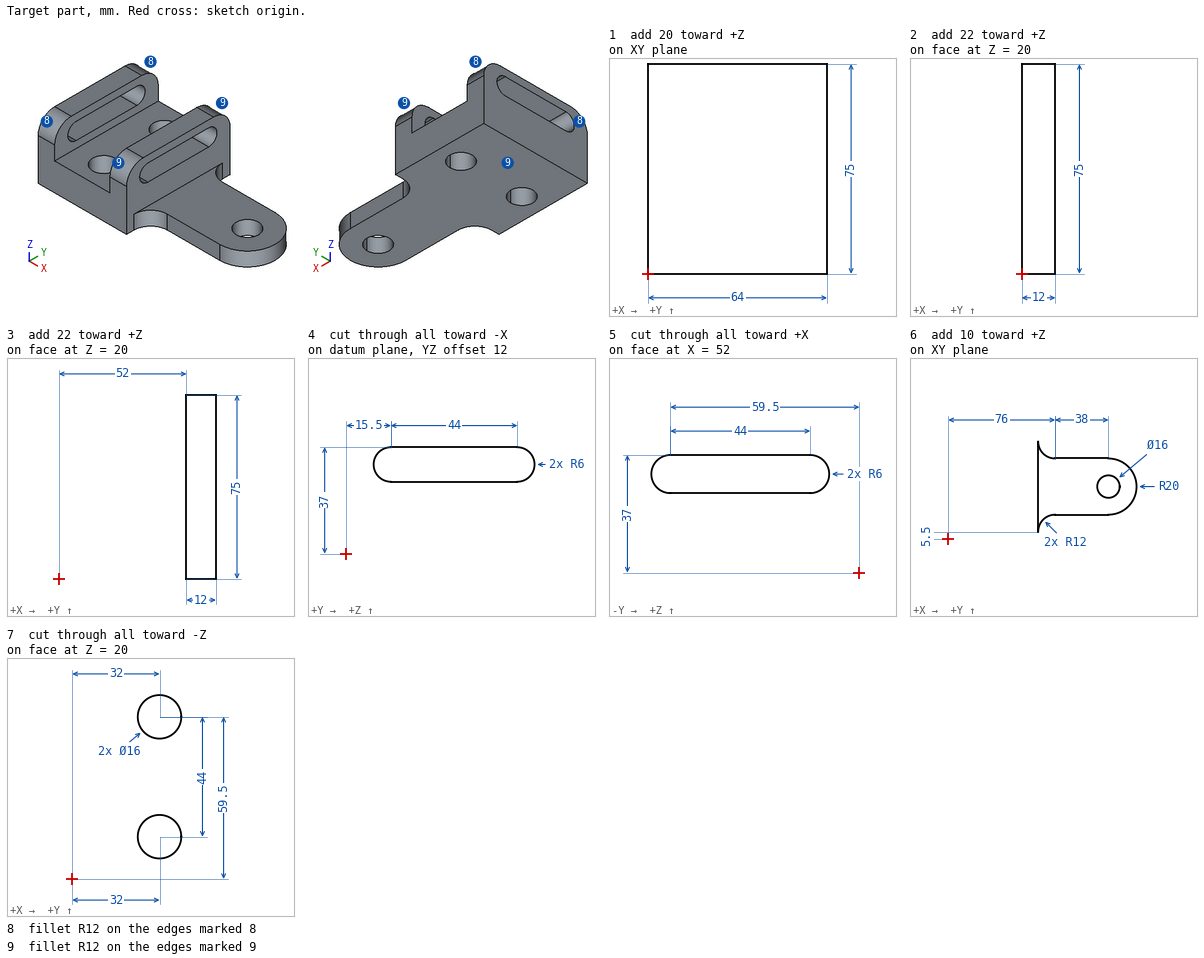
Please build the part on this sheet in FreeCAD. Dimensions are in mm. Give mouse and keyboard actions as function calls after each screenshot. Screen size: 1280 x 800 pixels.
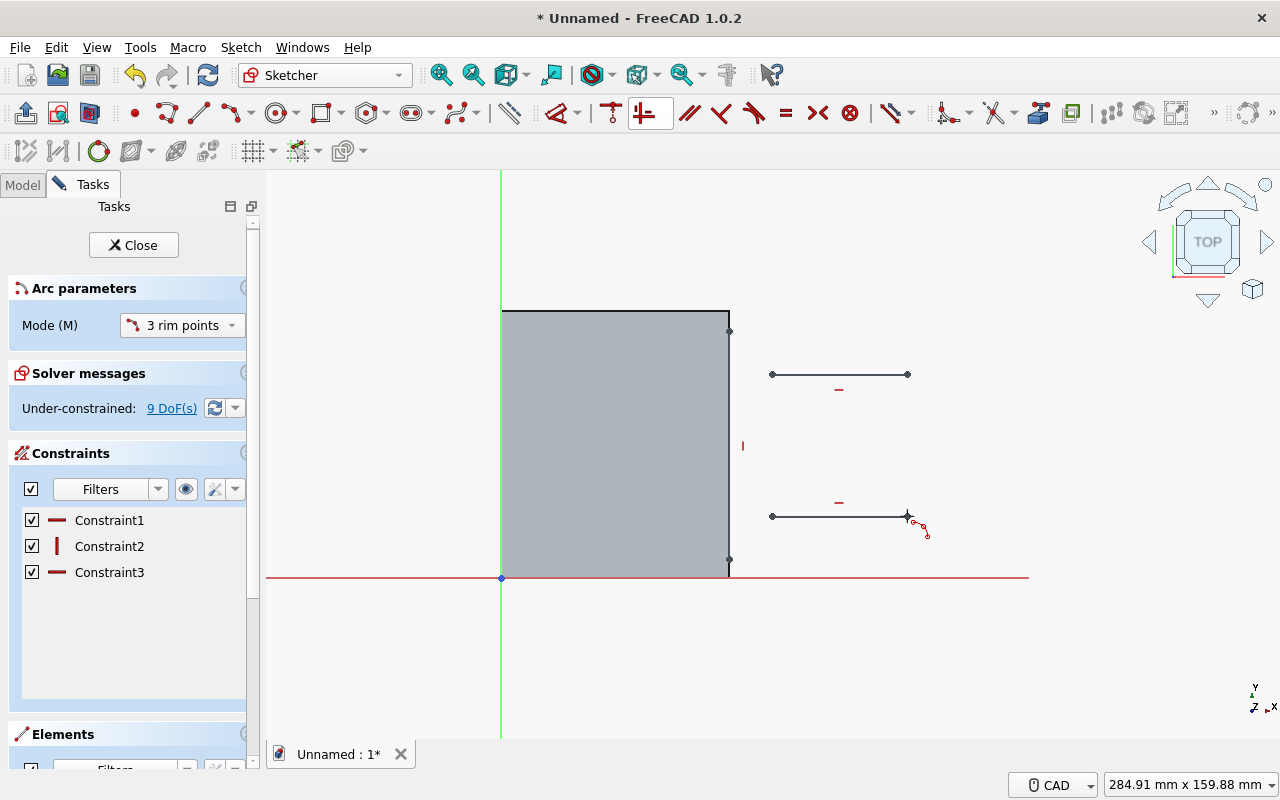
click(772, 375)
click(729, 332)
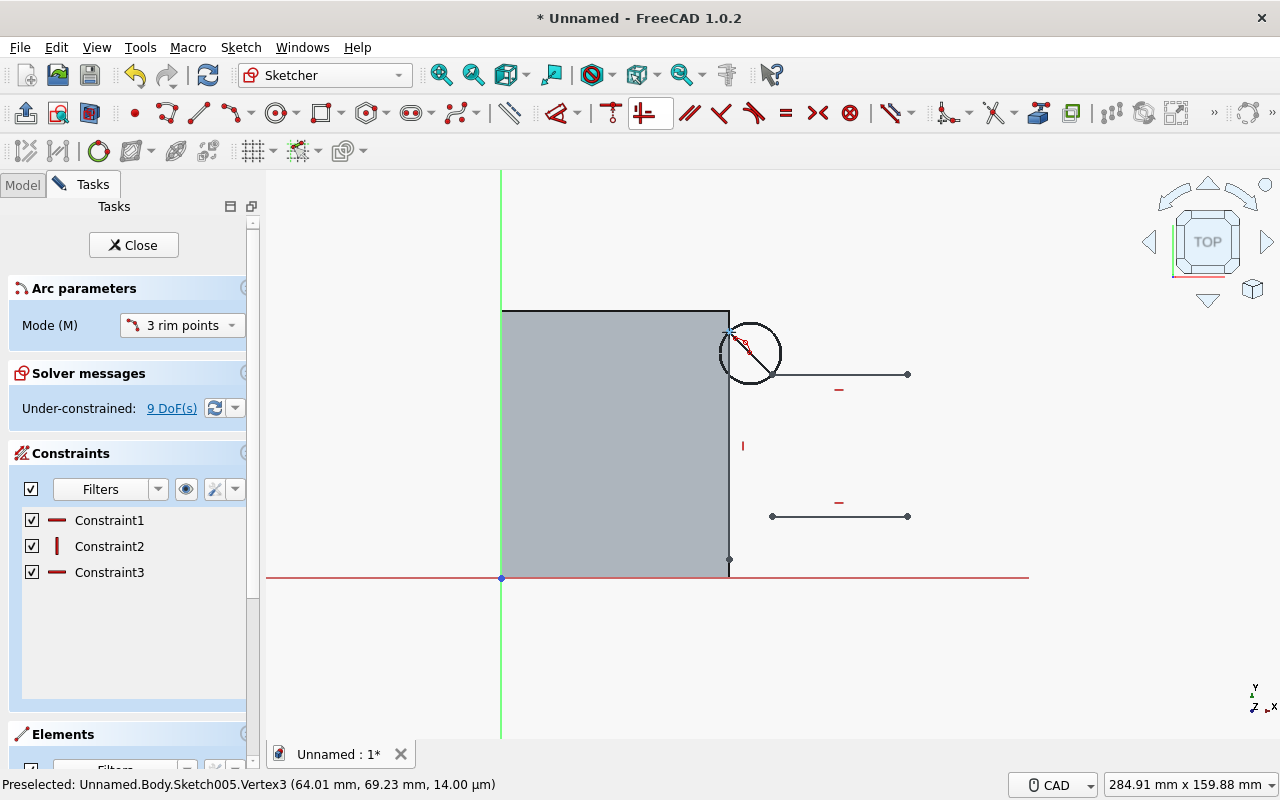
scroll(741, 361, up, 2)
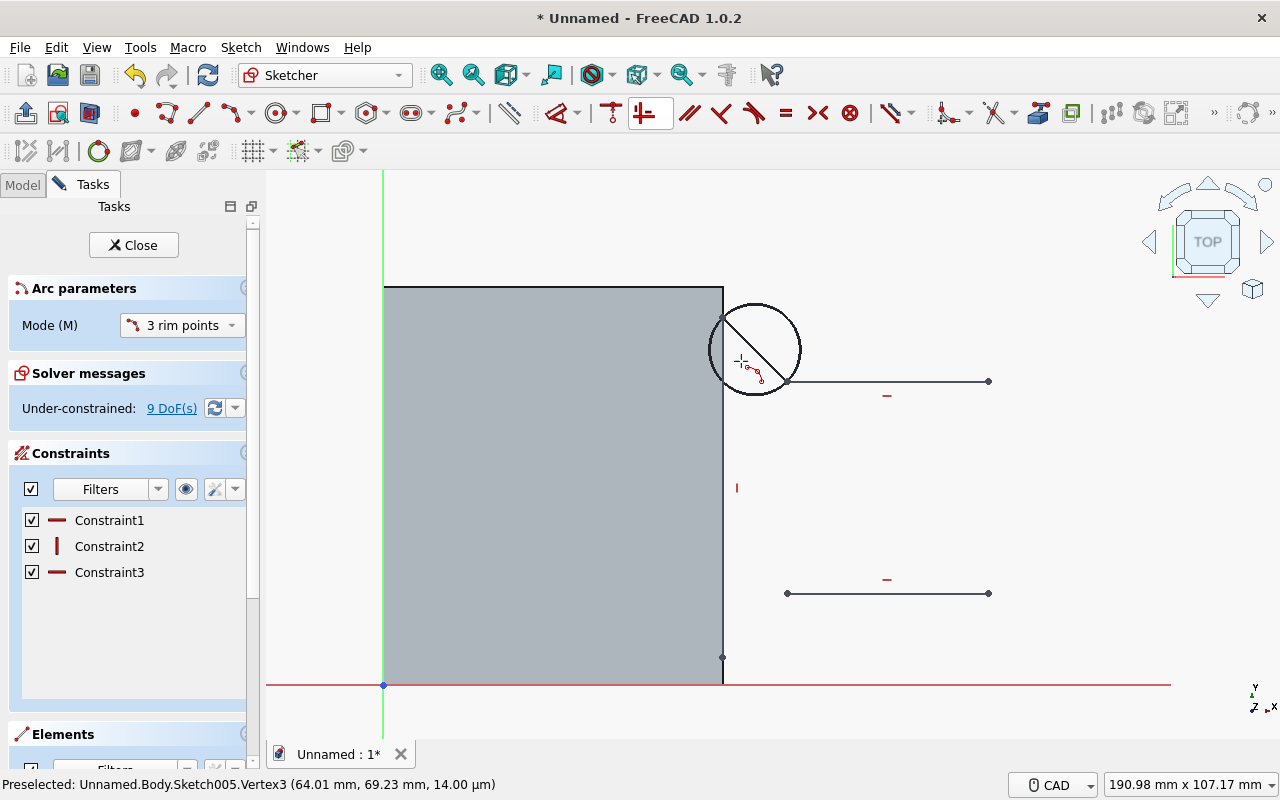
click(741, 361)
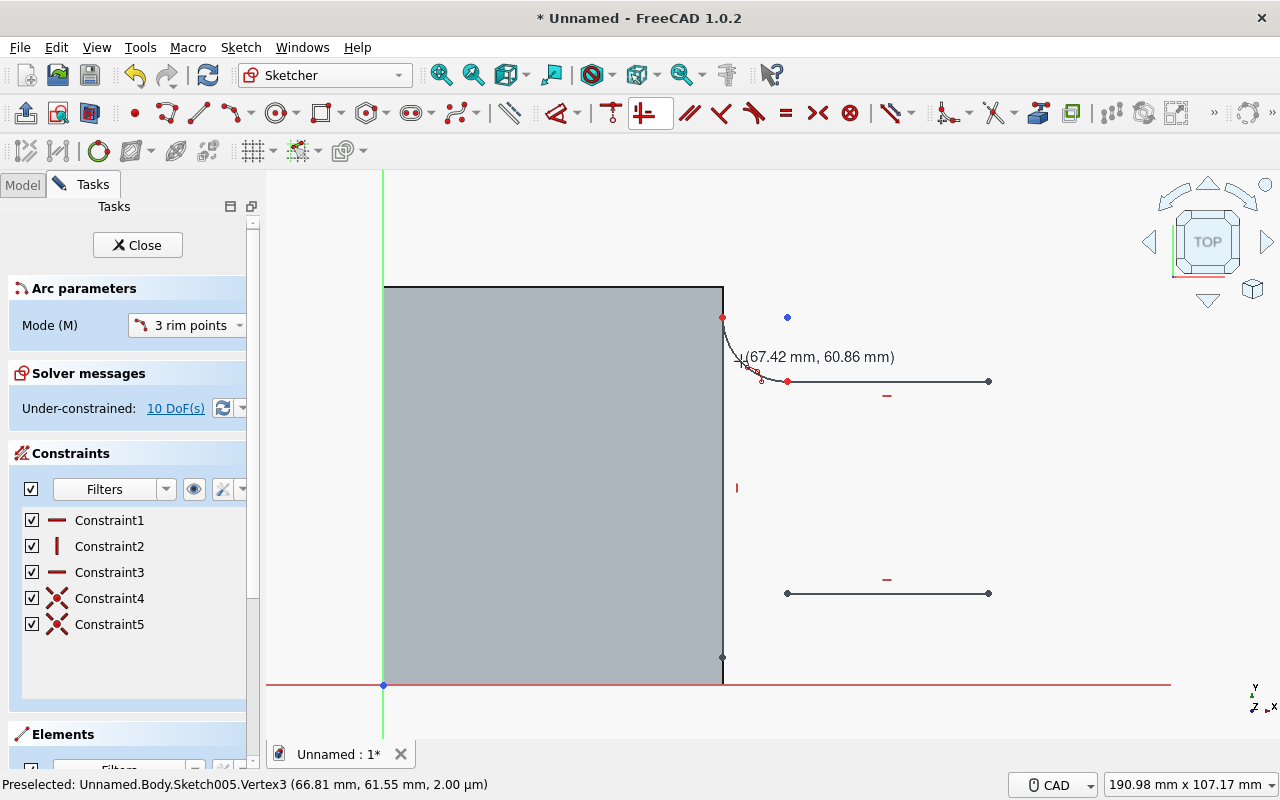
click(723, 658)
click(787, 594)
click(741, 611)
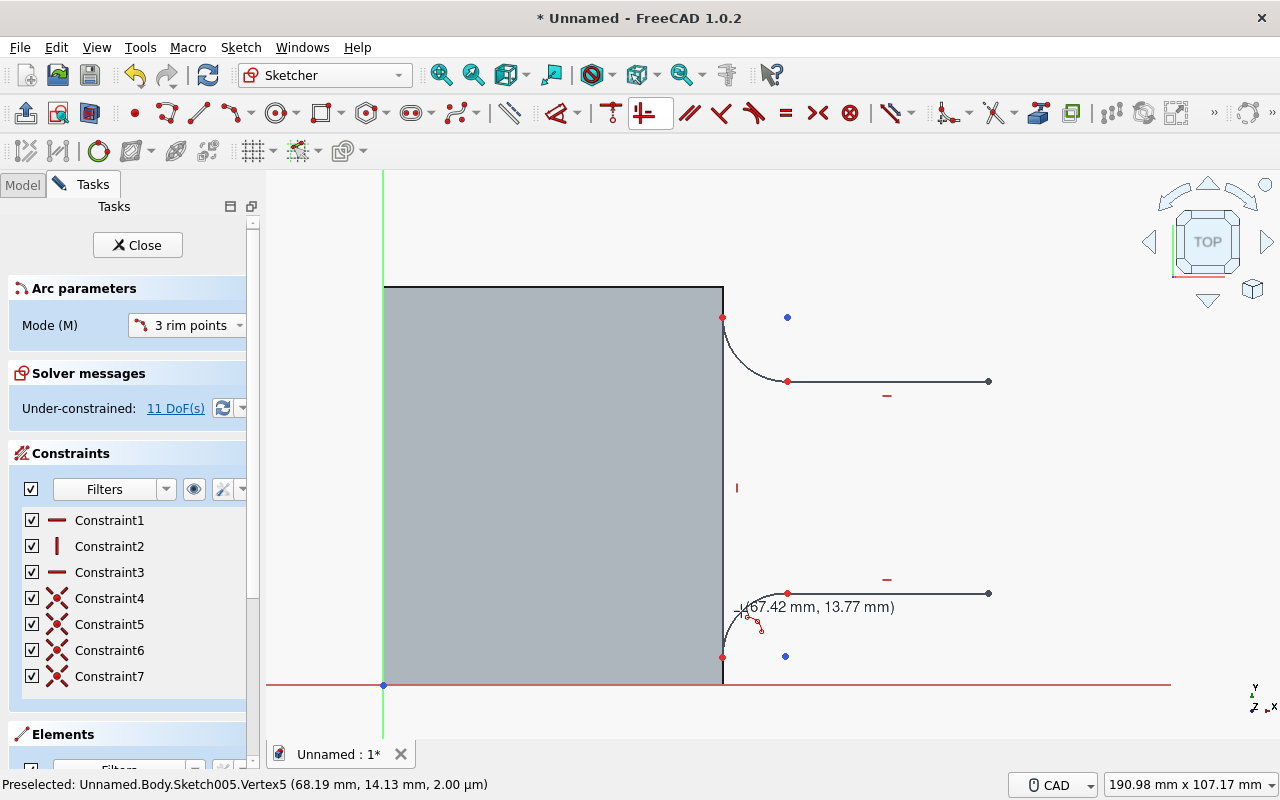
click(988, 594)
click(988, 382)
click(1094, 486)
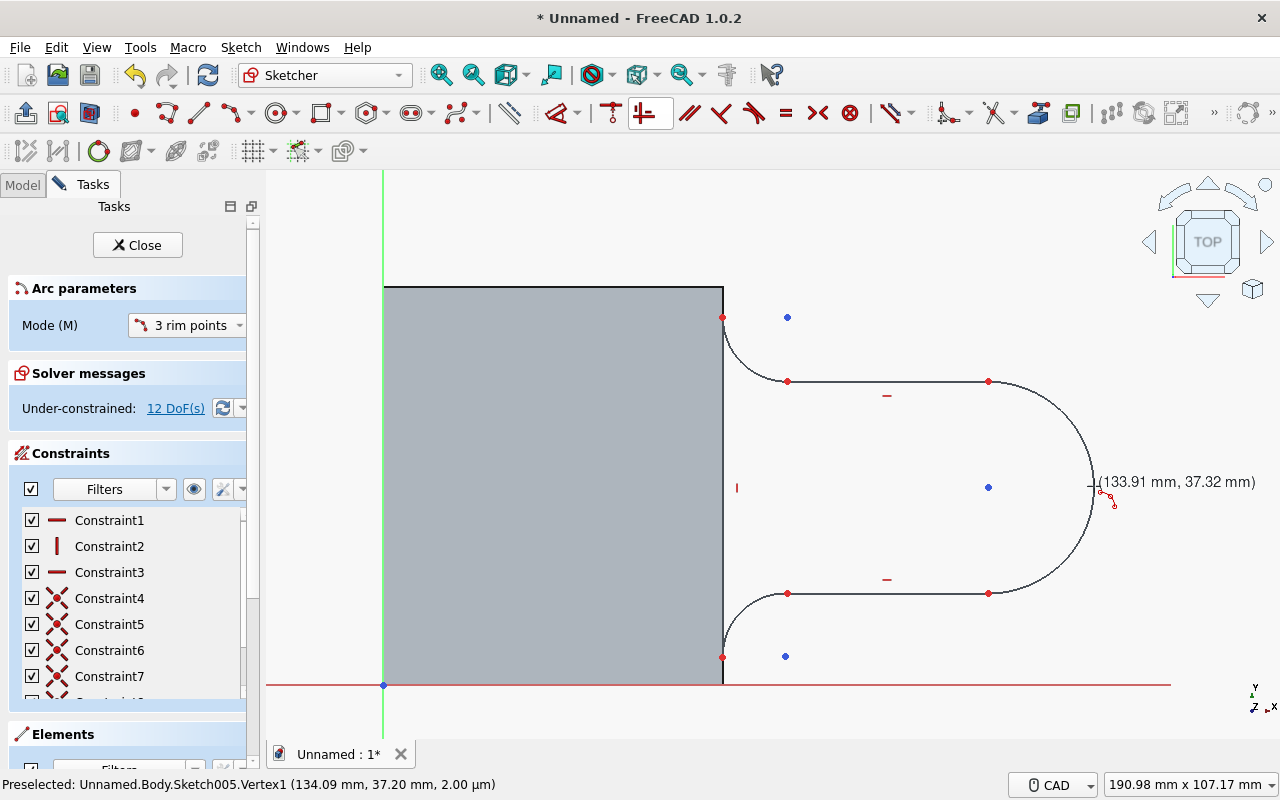
click(276, 114)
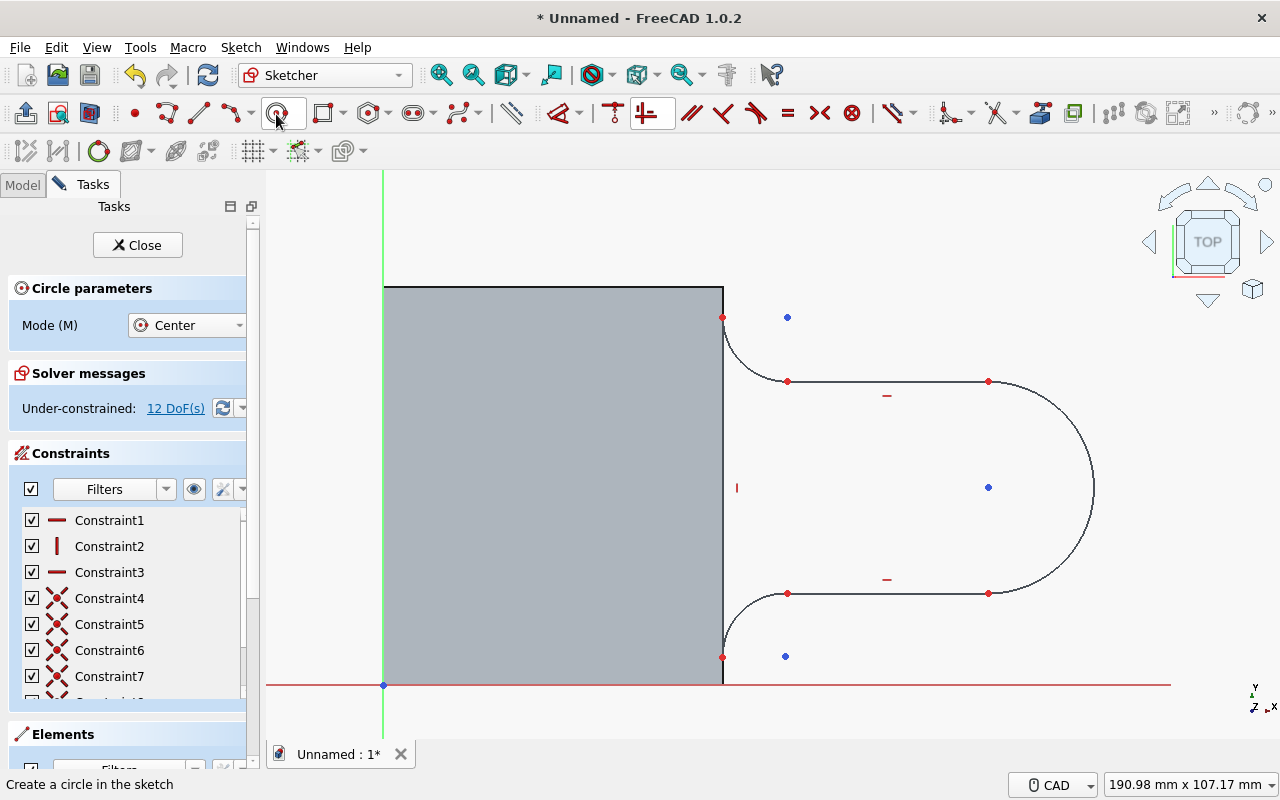
click(988, 486)
click(1018, 456)
key(Escape)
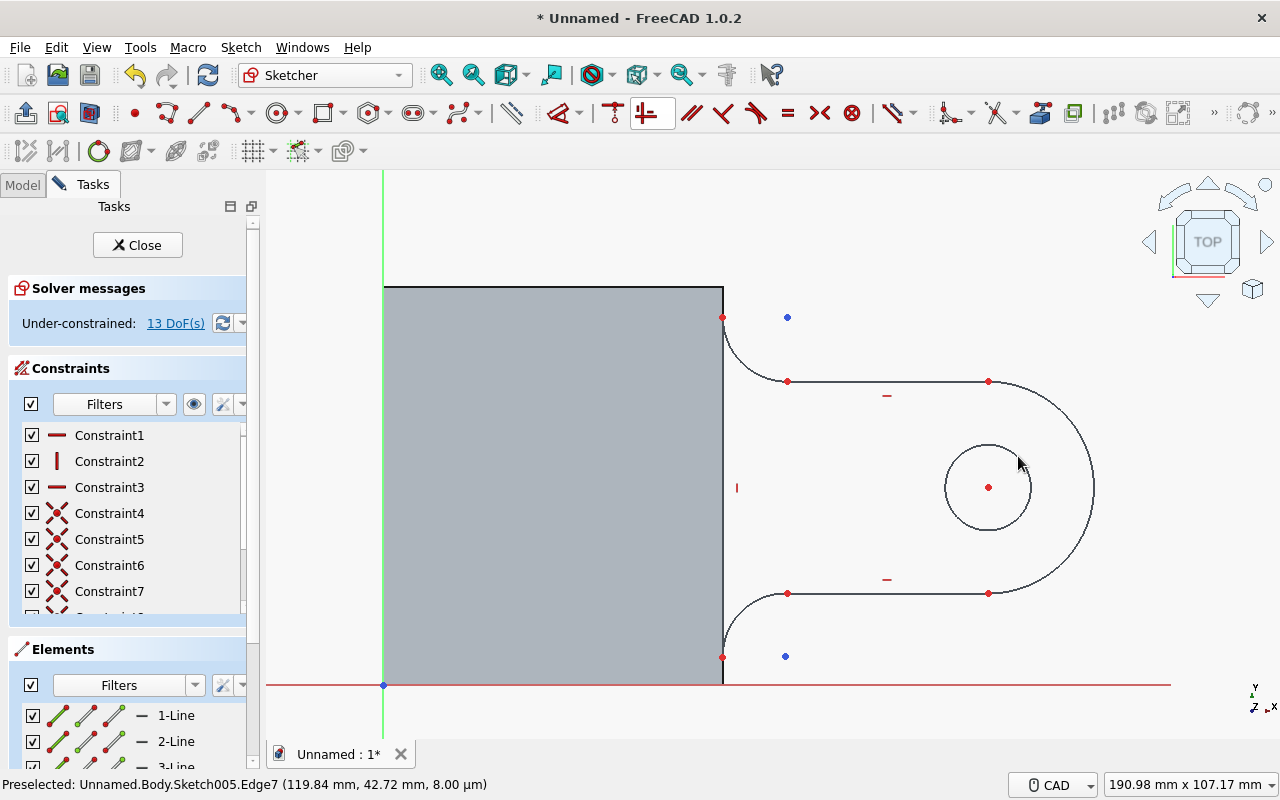
click(928, 382)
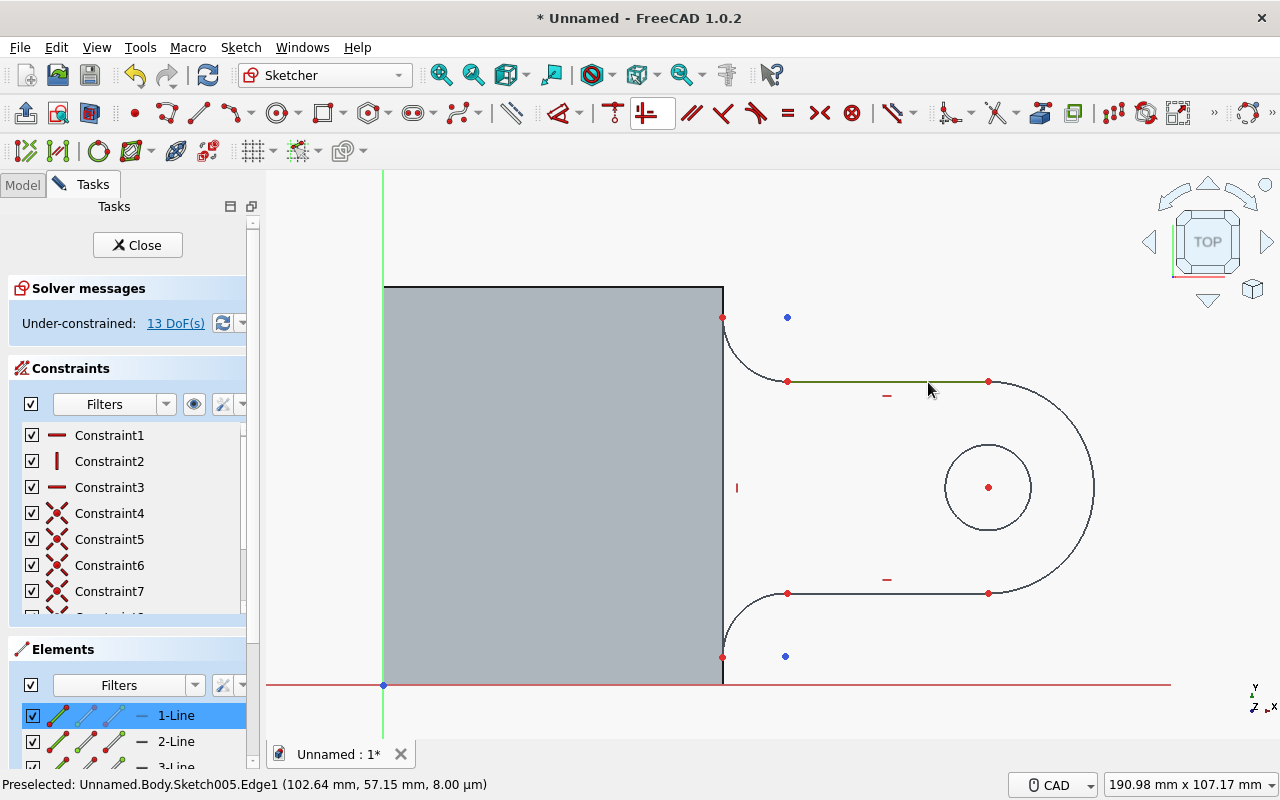
click(758, 375)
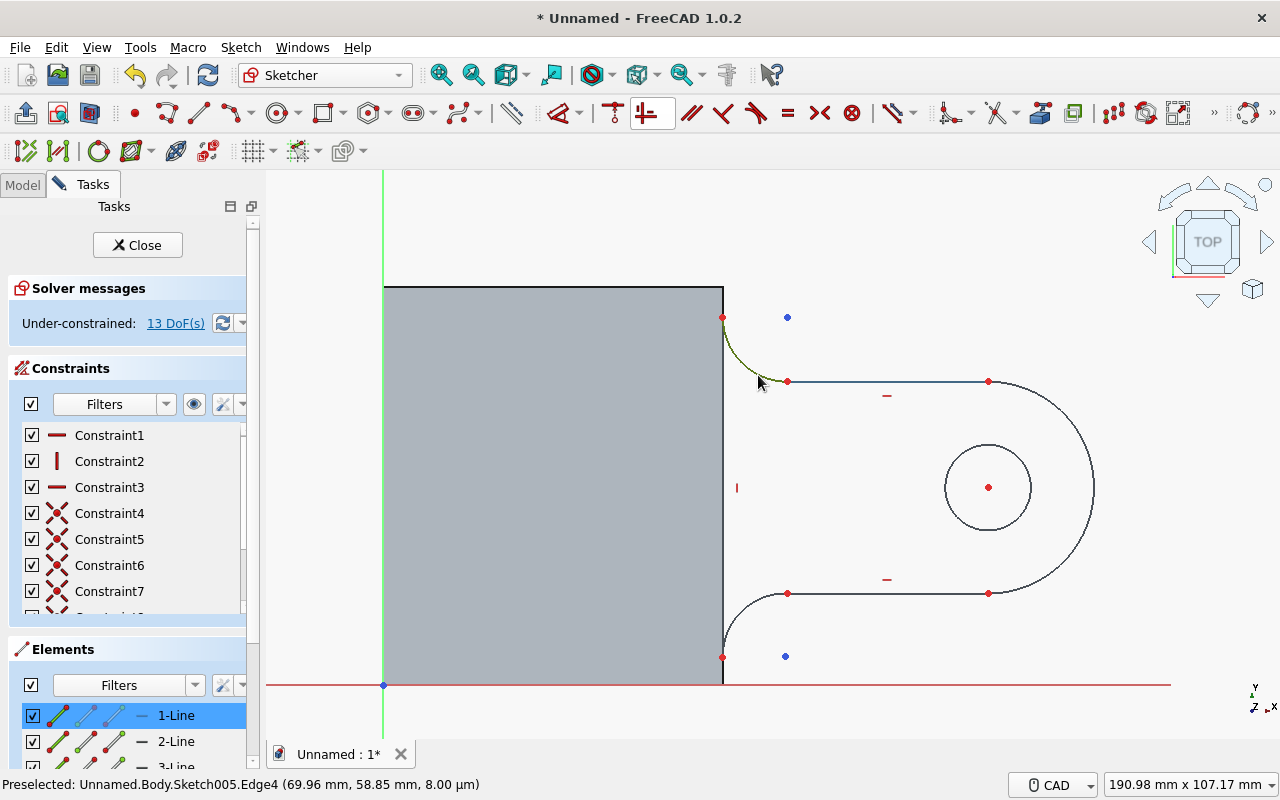
click(756, 114)